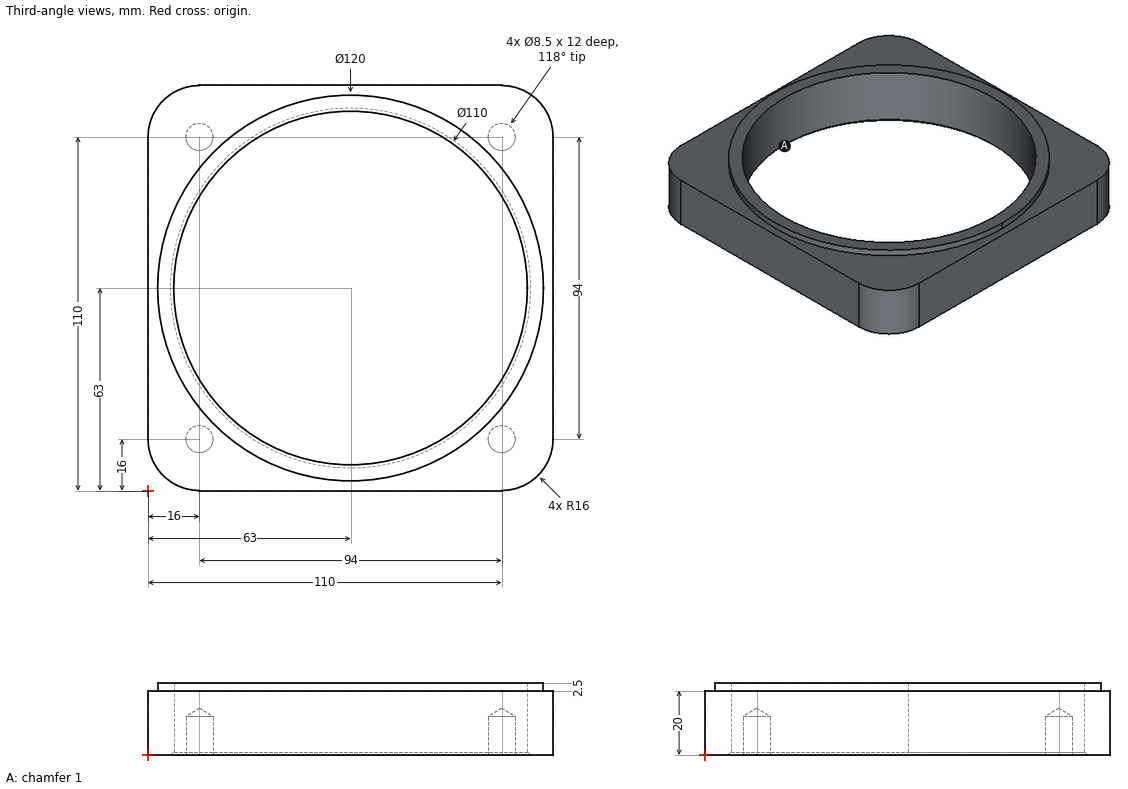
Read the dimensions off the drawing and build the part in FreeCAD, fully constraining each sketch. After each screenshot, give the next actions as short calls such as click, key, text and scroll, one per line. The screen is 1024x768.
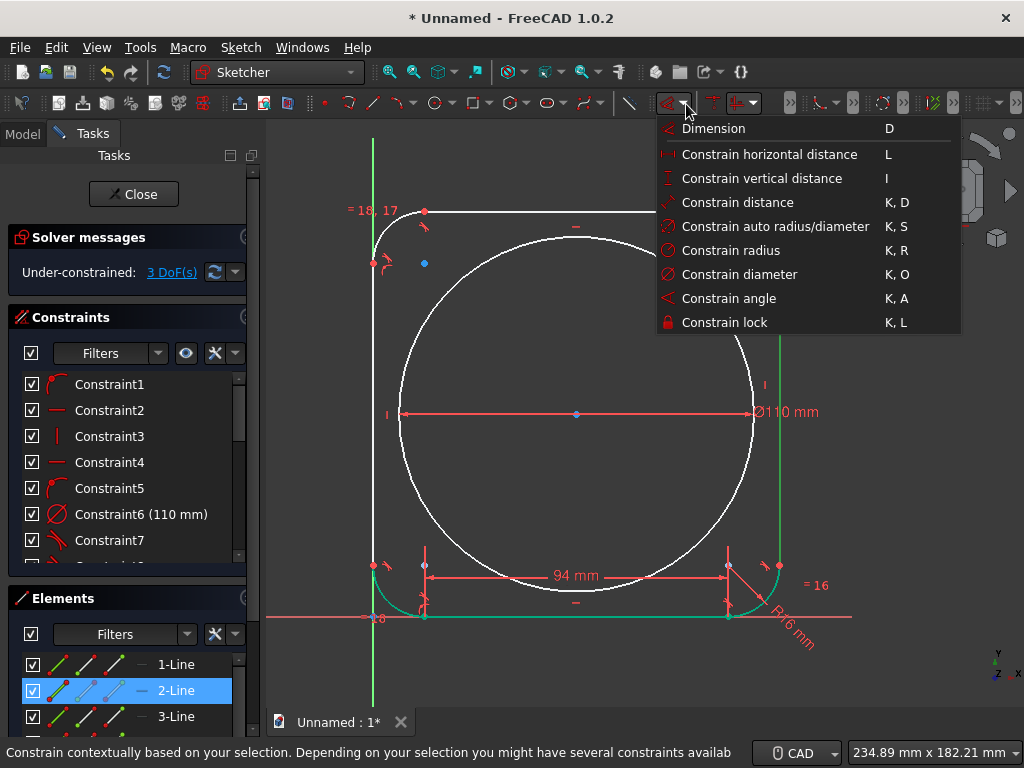
click(809, 178)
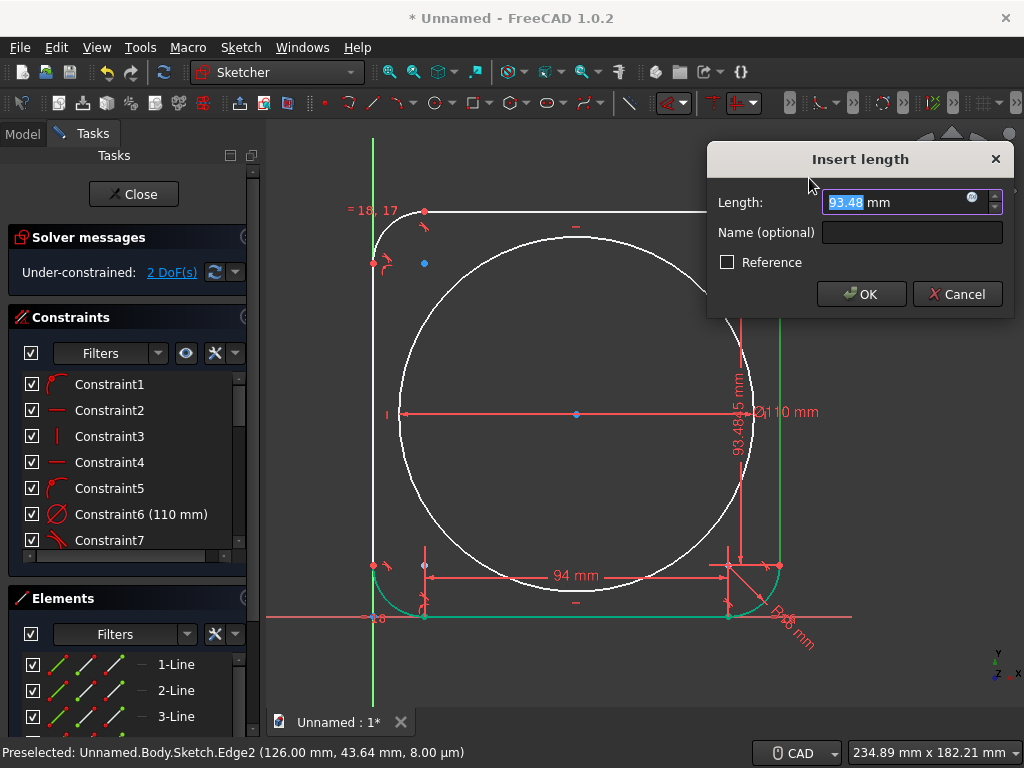
text(94)
key(Return)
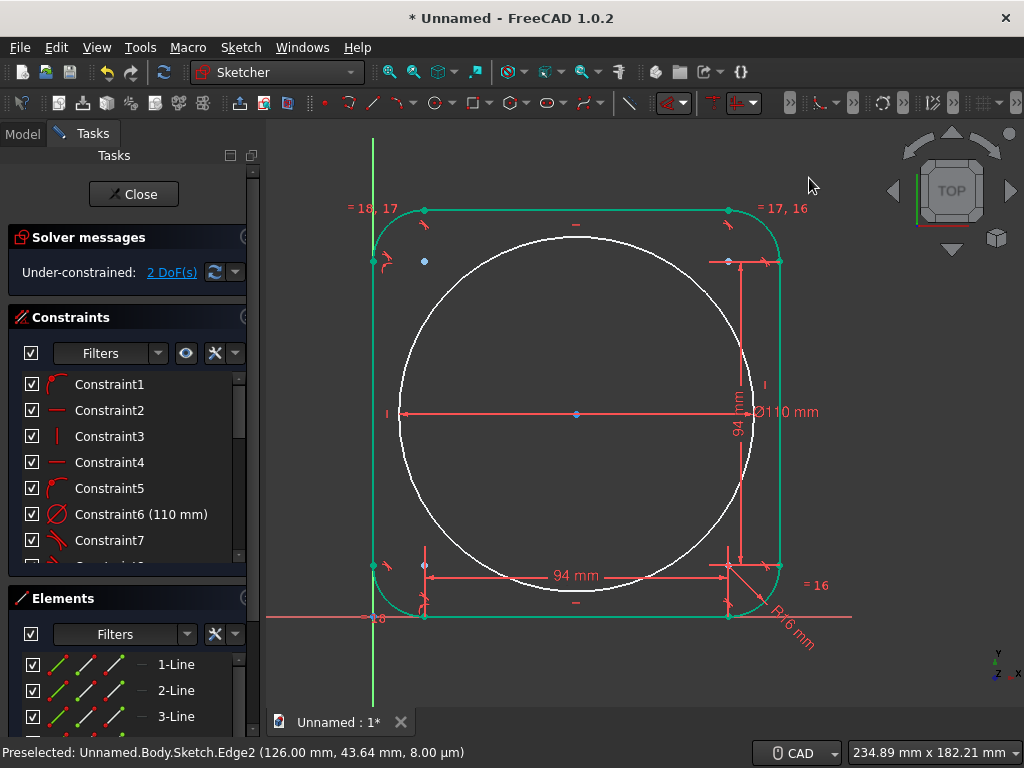
click(577, 414)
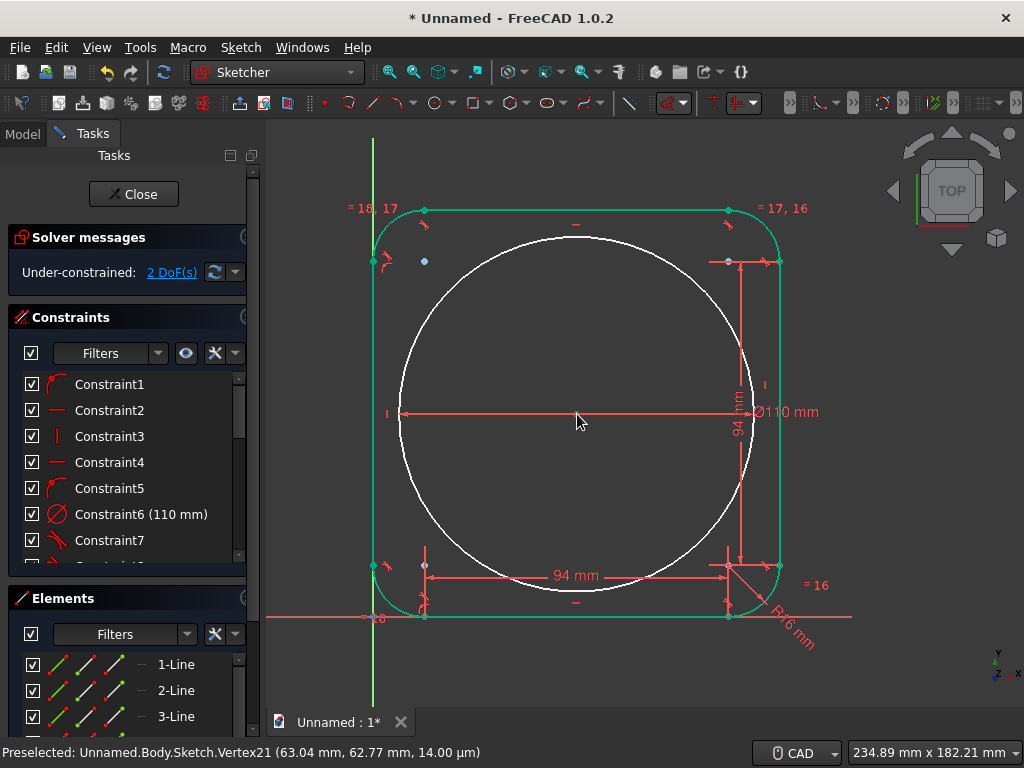
click(686, 104)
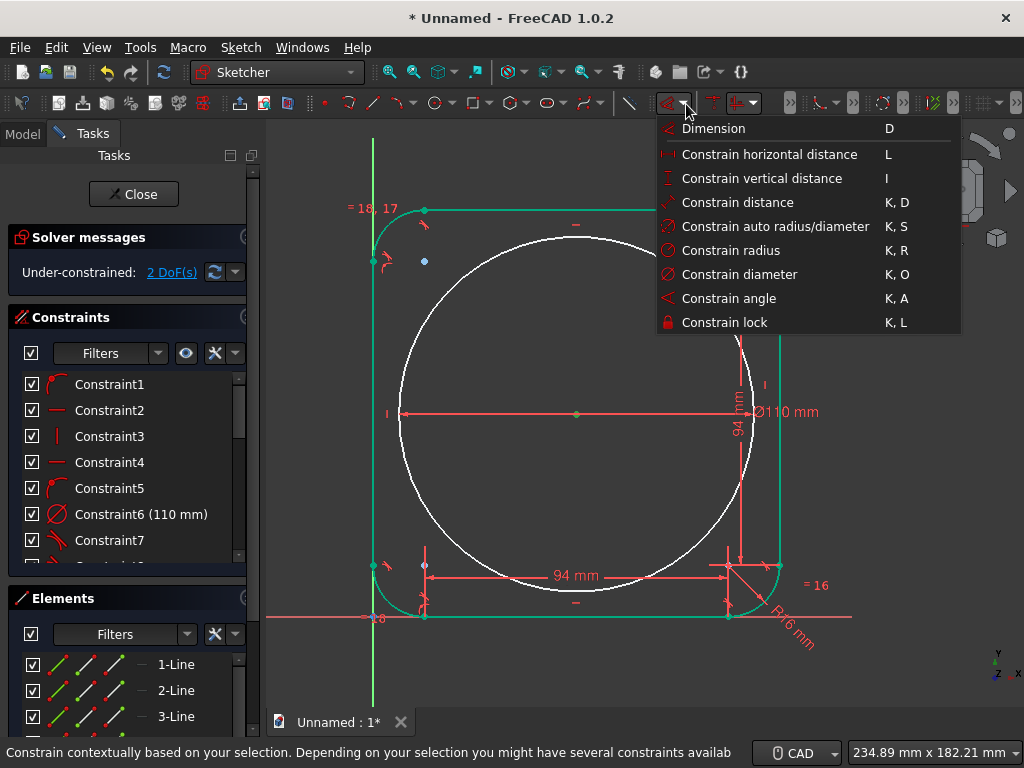
click(809, 154)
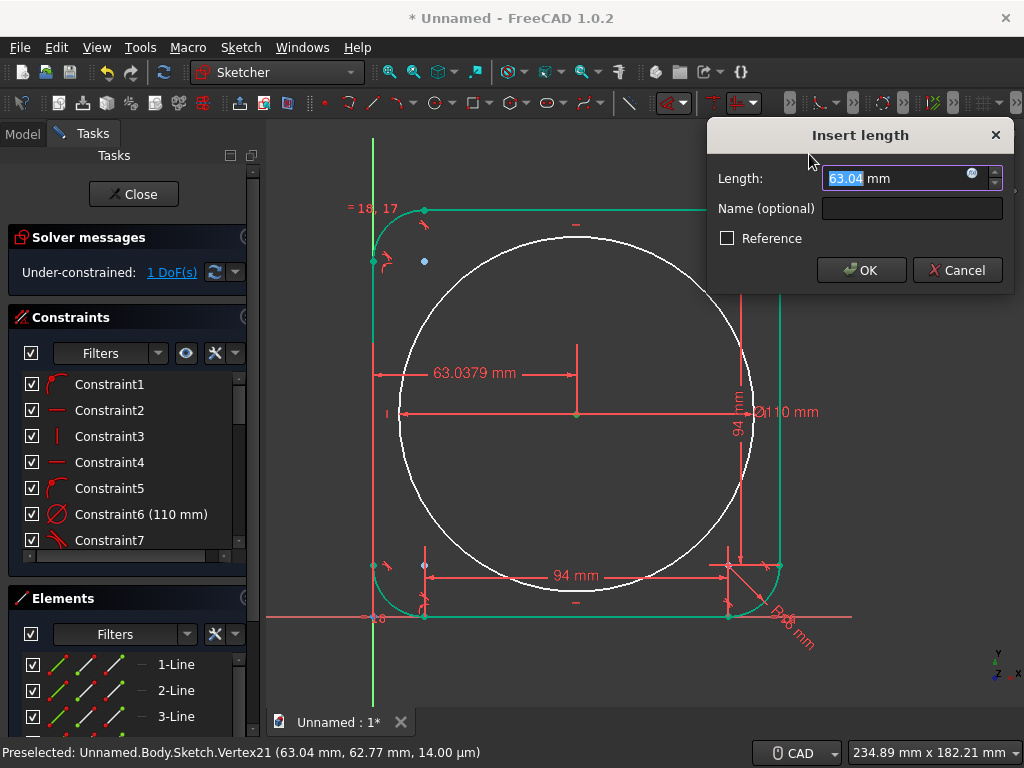
text(63)
key(Return)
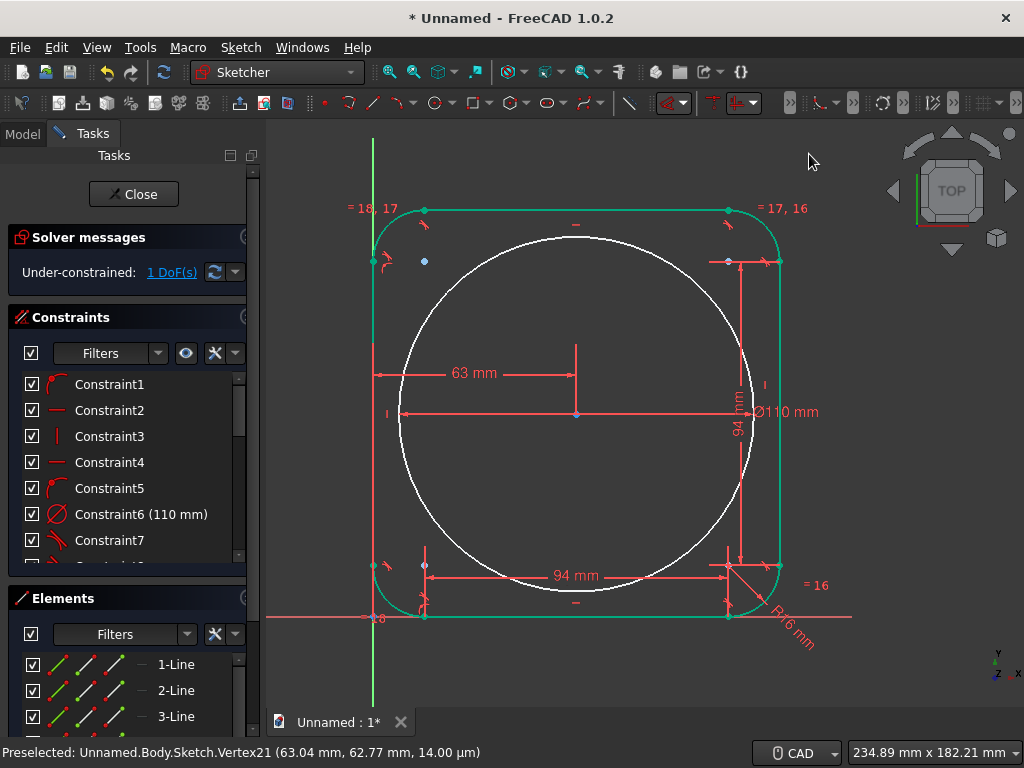
click(576, 414)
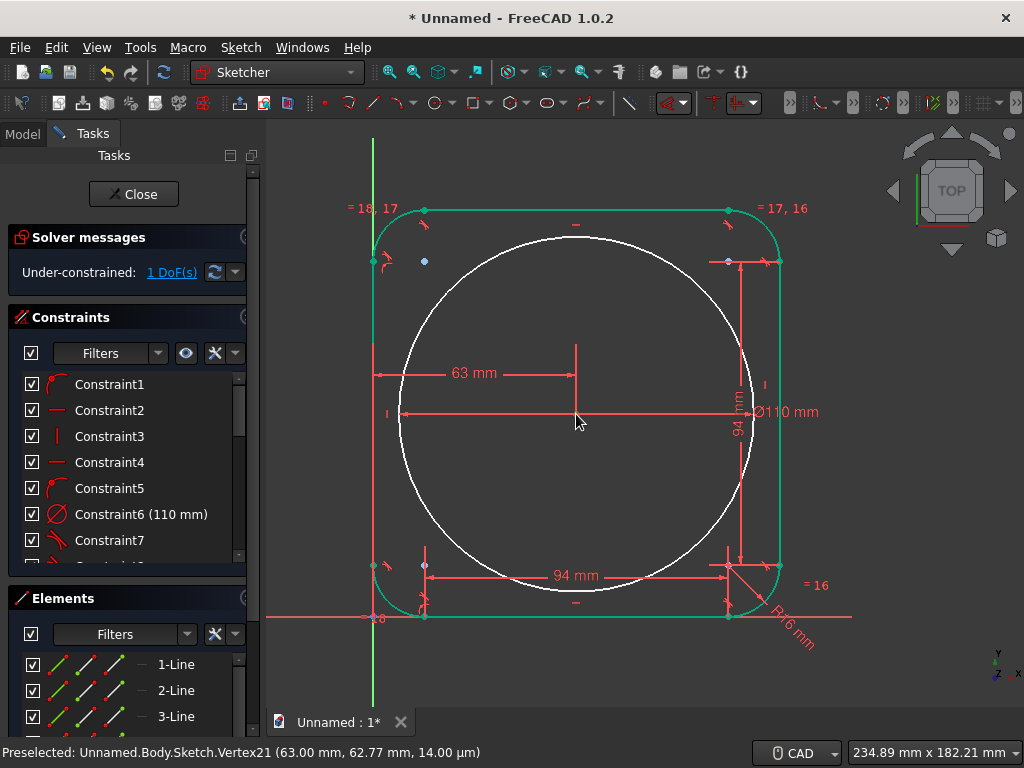
click(686, 104)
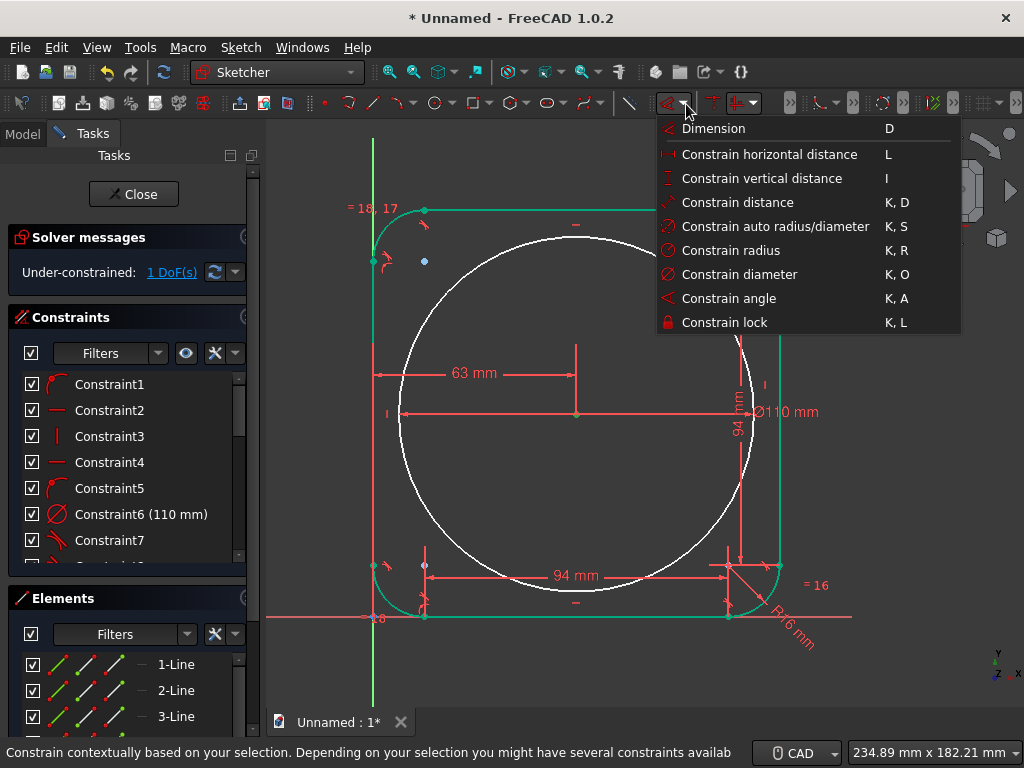
click(809, 178)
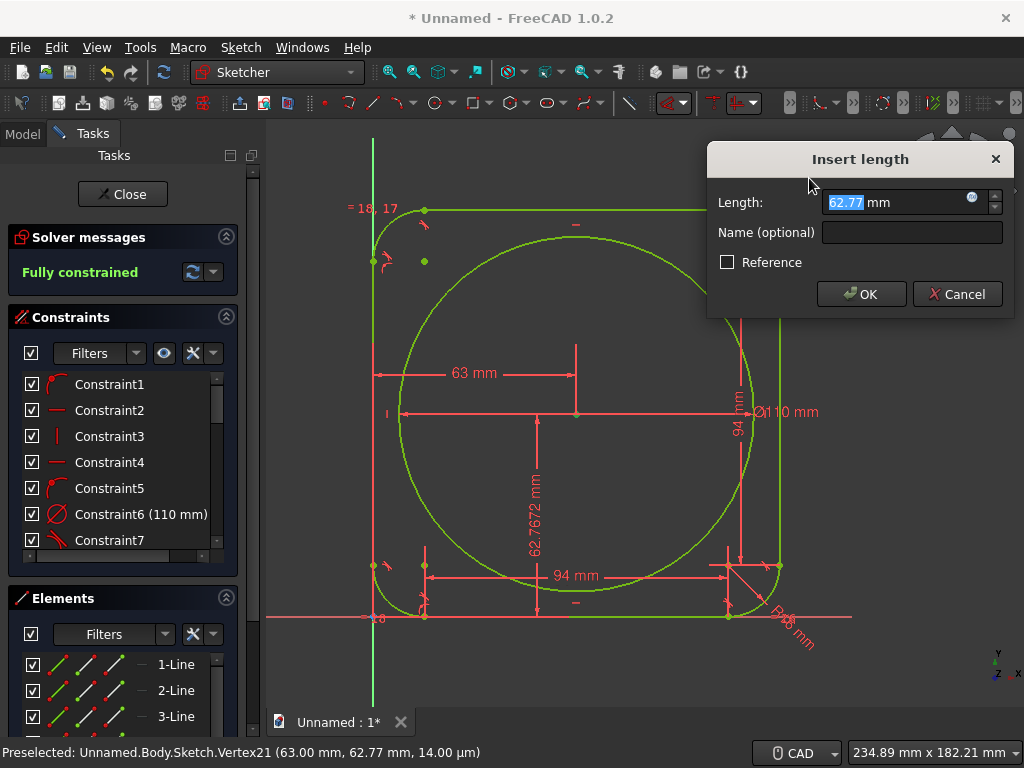
text(63)
key(Return)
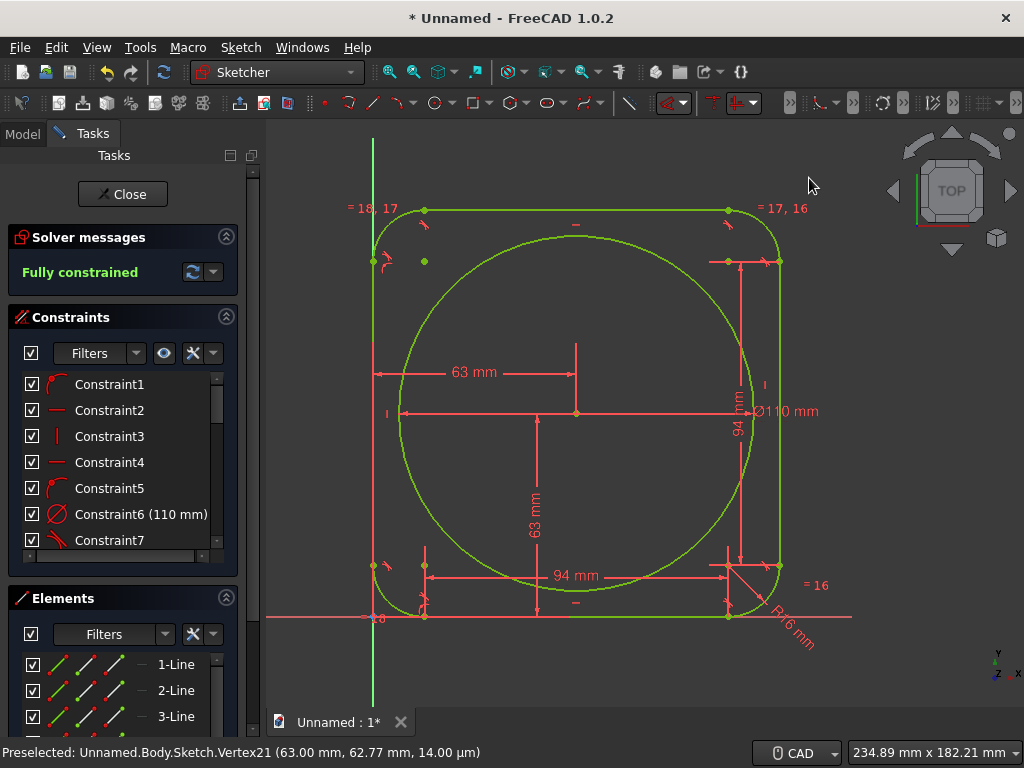
click(123, 194)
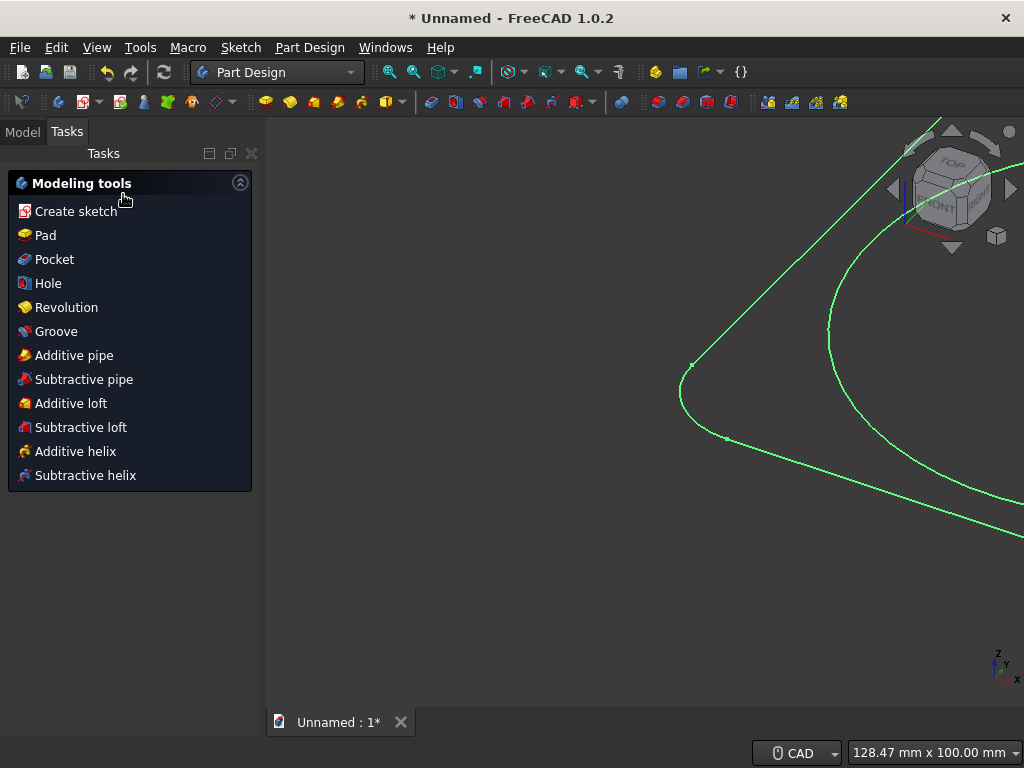
click(266, 102)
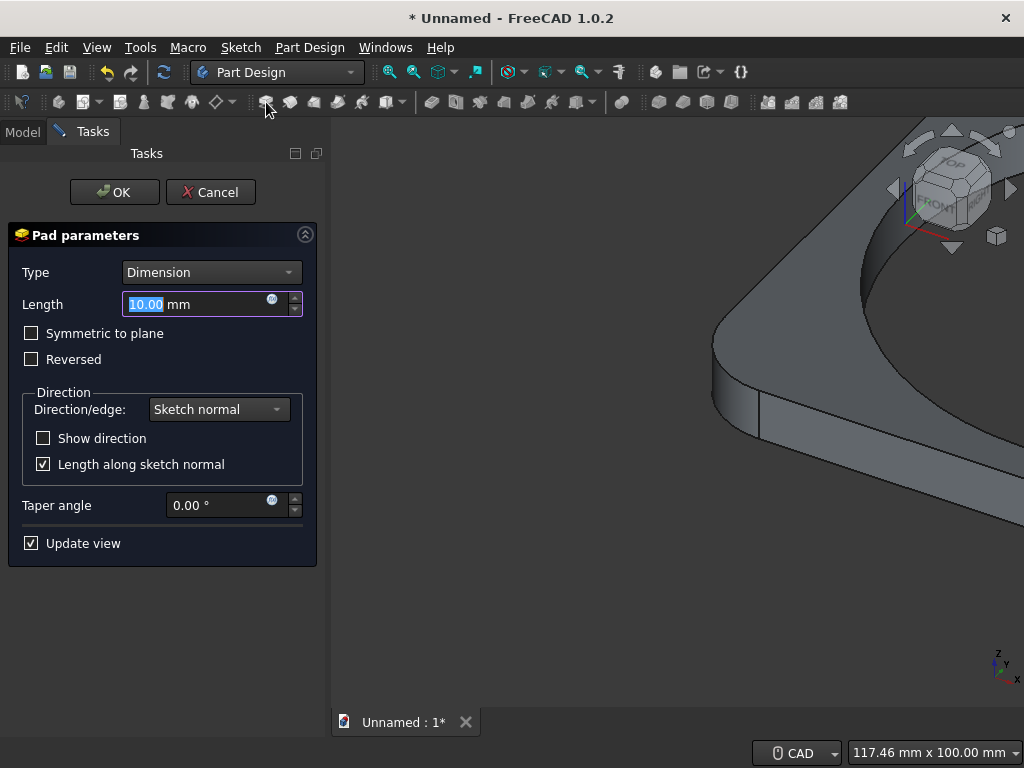
text(20)
key(Tab)